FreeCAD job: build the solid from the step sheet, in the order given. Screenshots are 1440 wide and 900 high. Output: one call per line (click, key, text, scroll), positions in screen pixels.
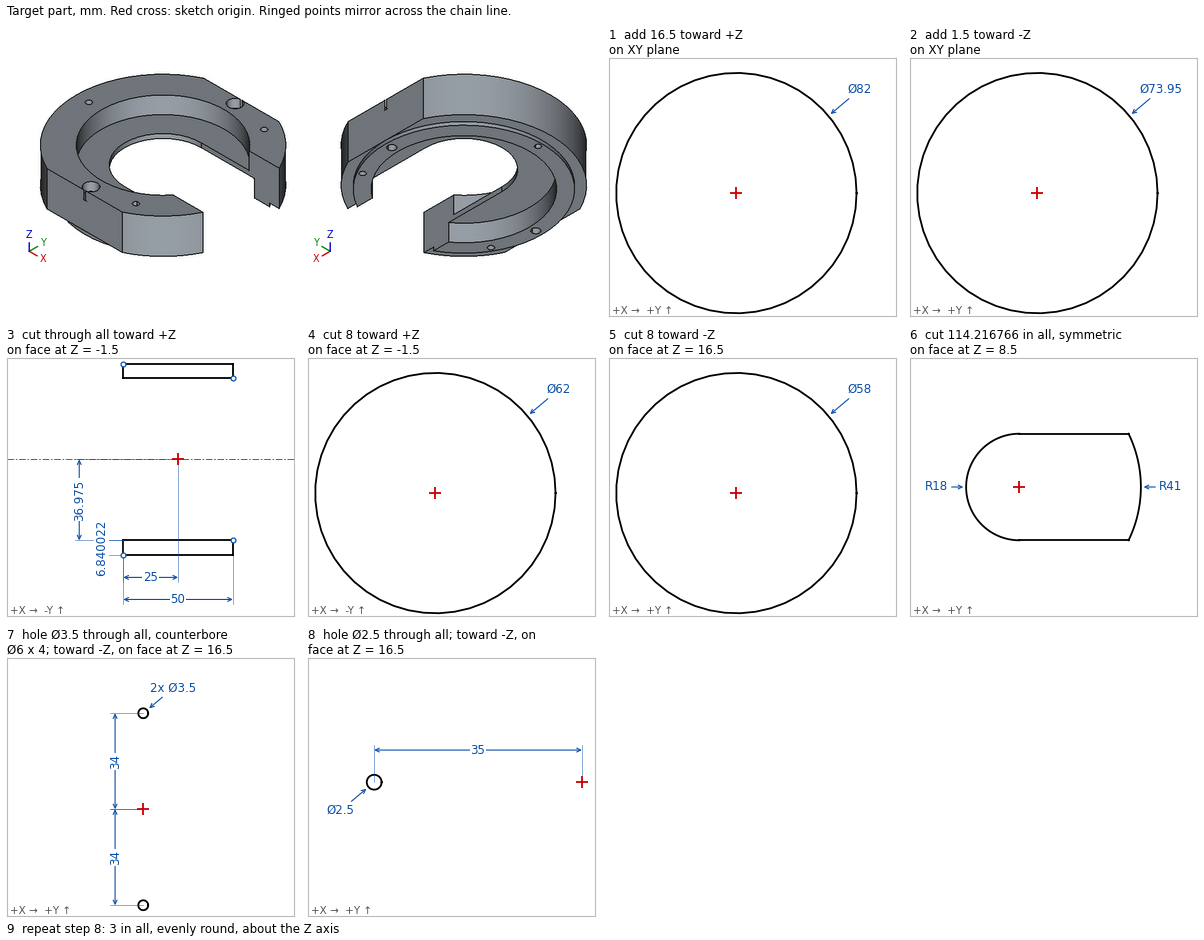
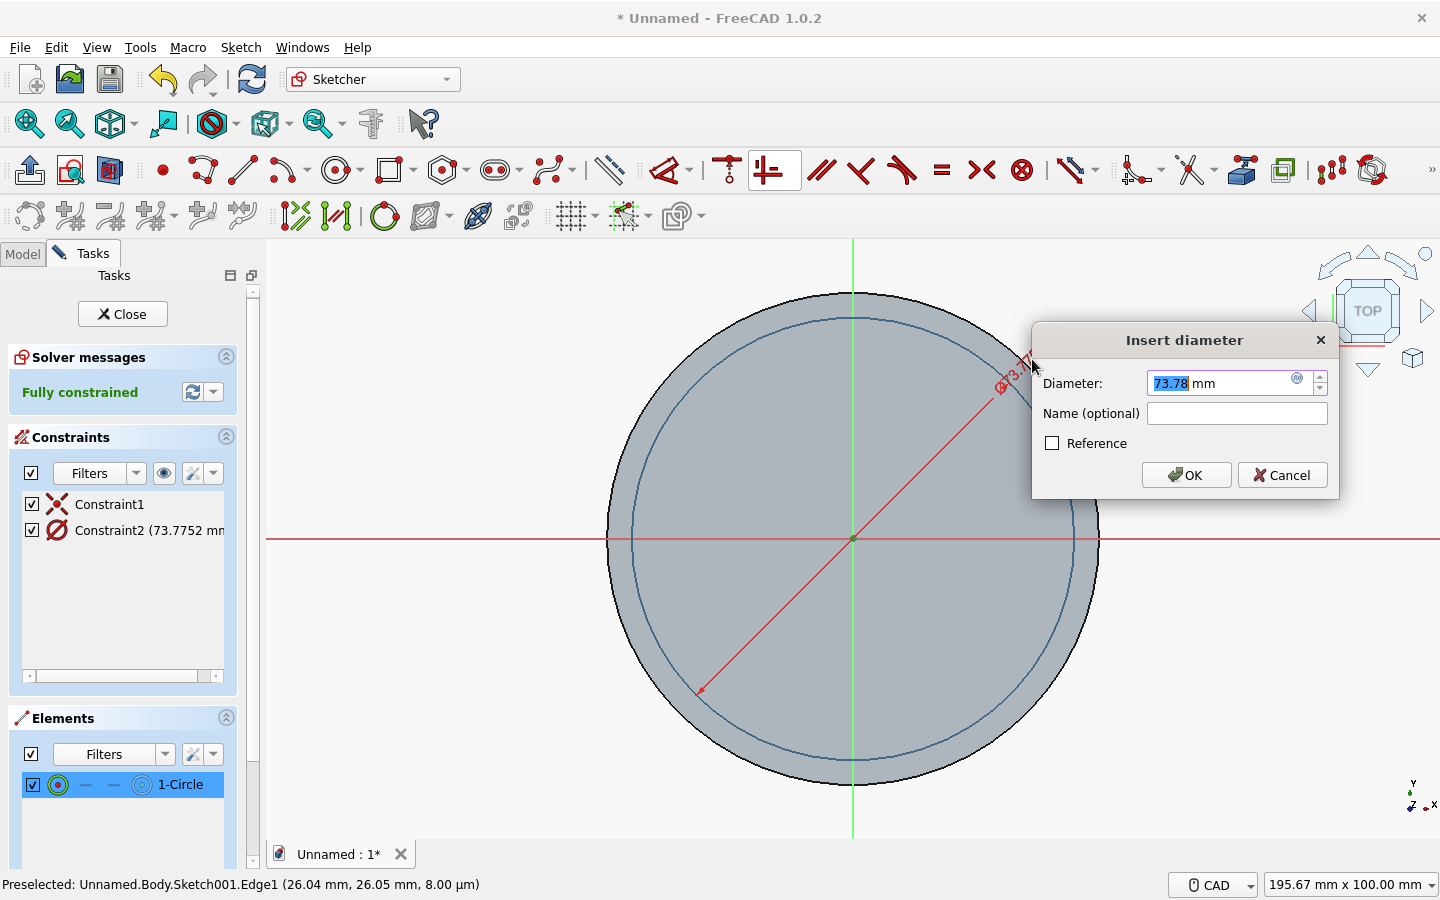
text(73.95)
key(Return)
key(Escape)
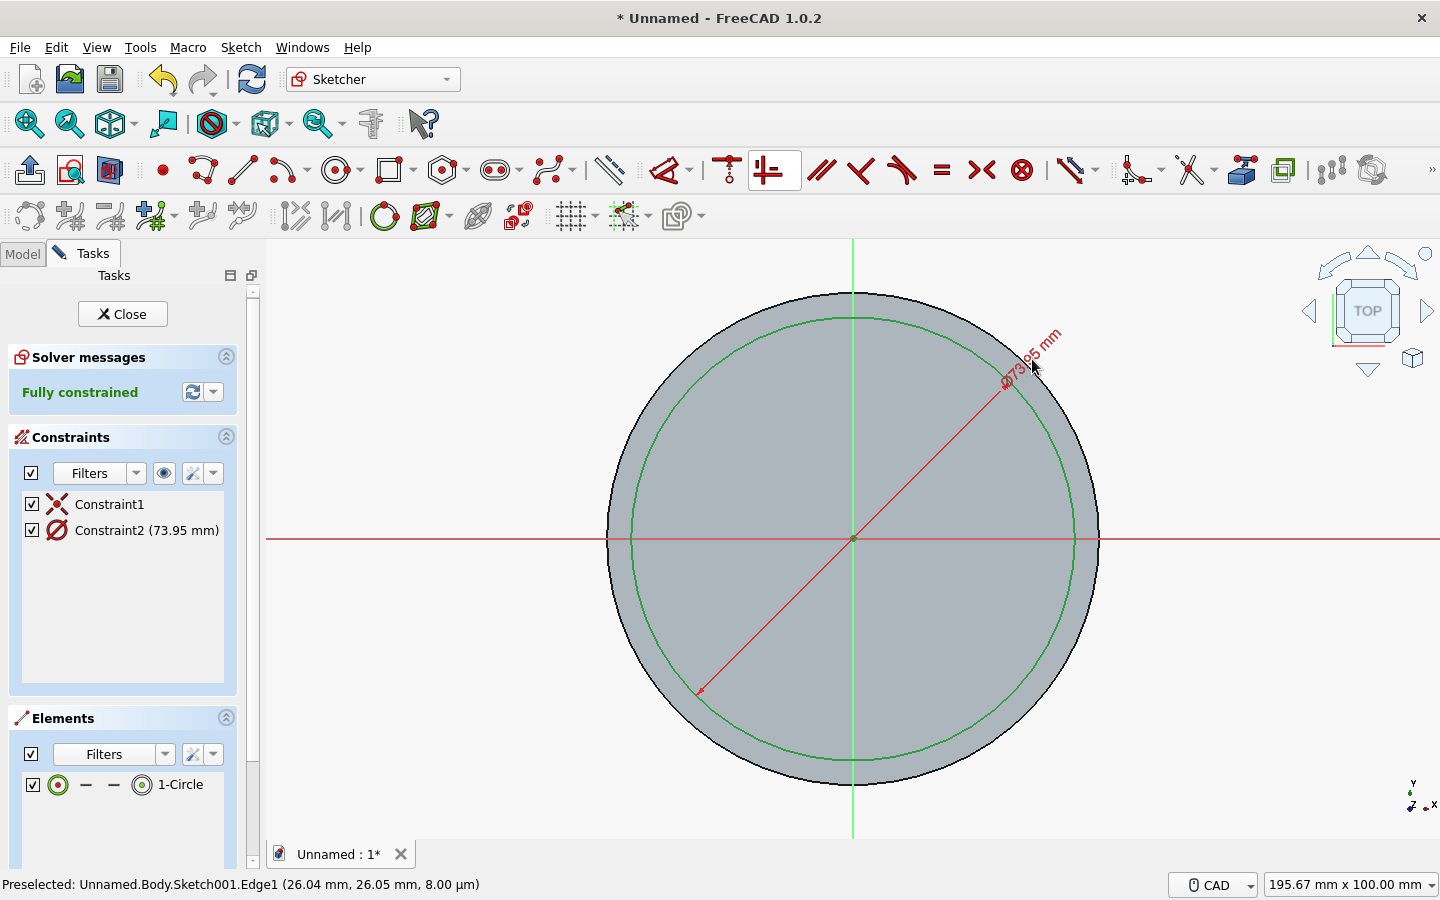
click(123, 314)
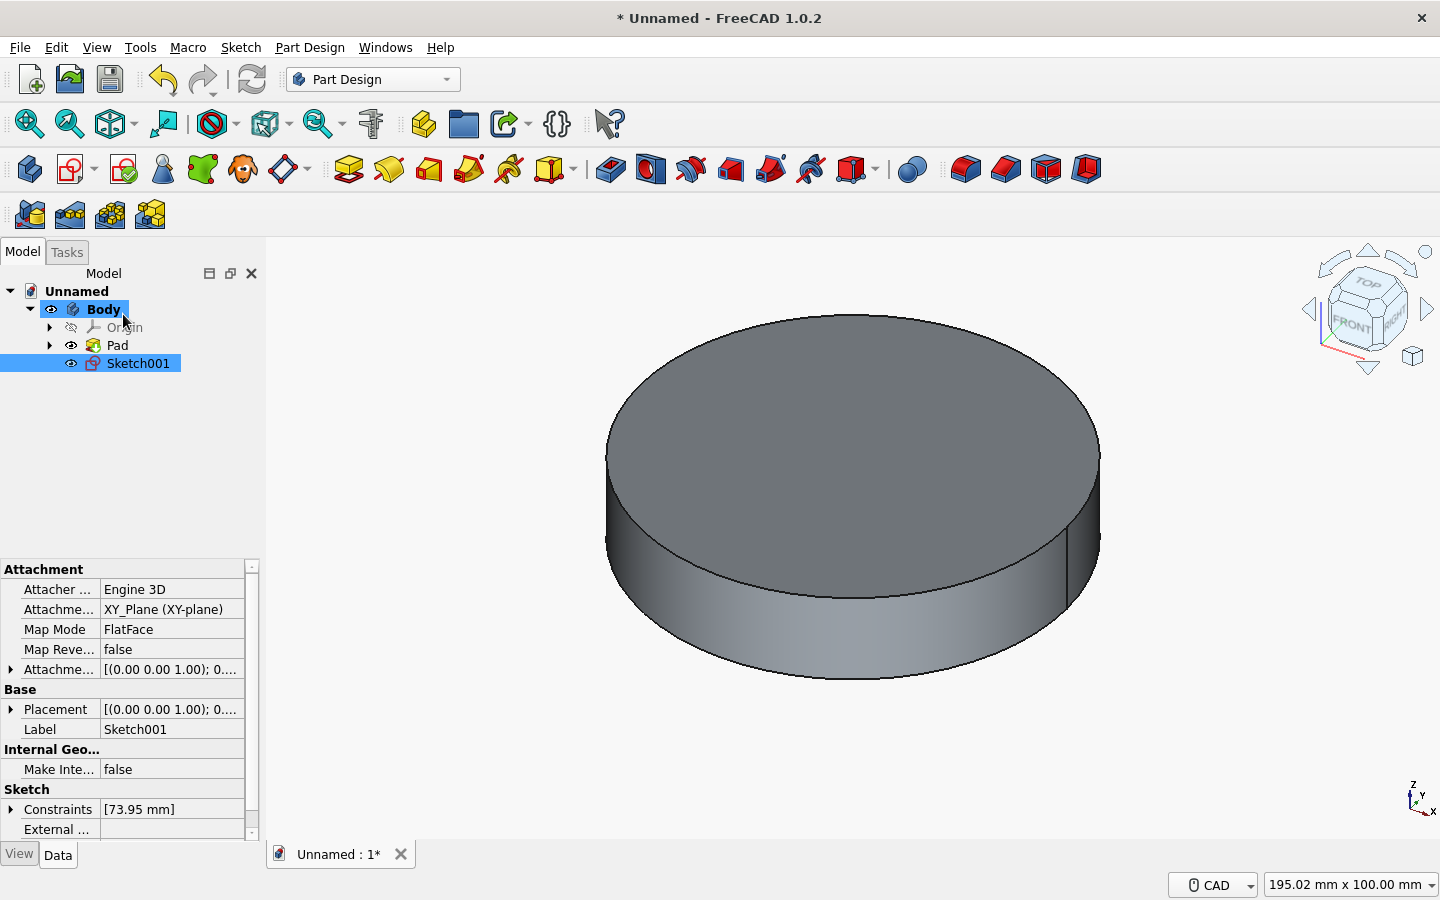
click(350, 170)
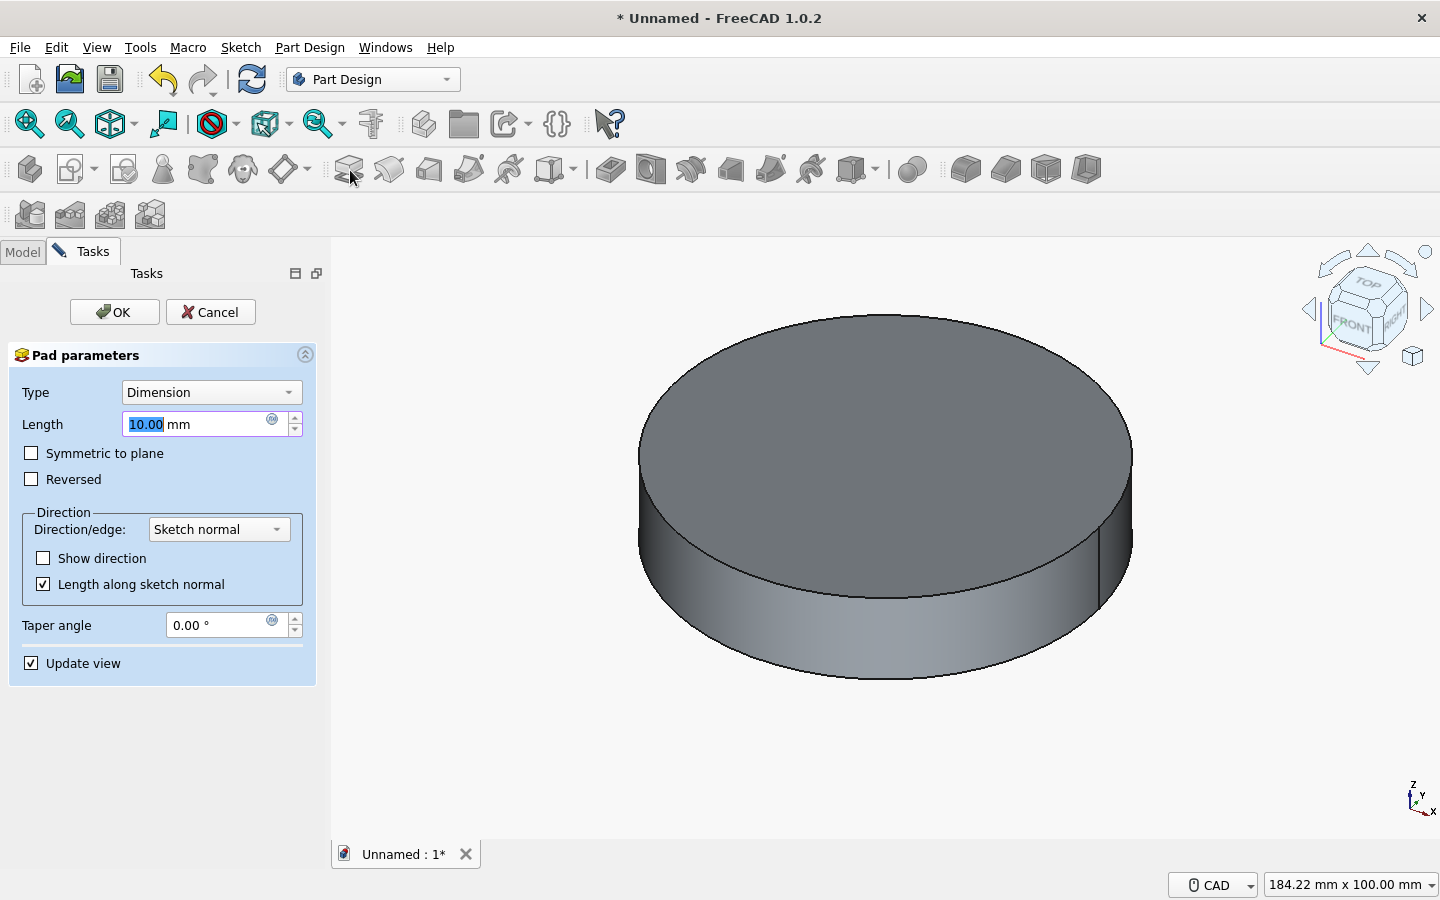
text(1.5)
key(Tab)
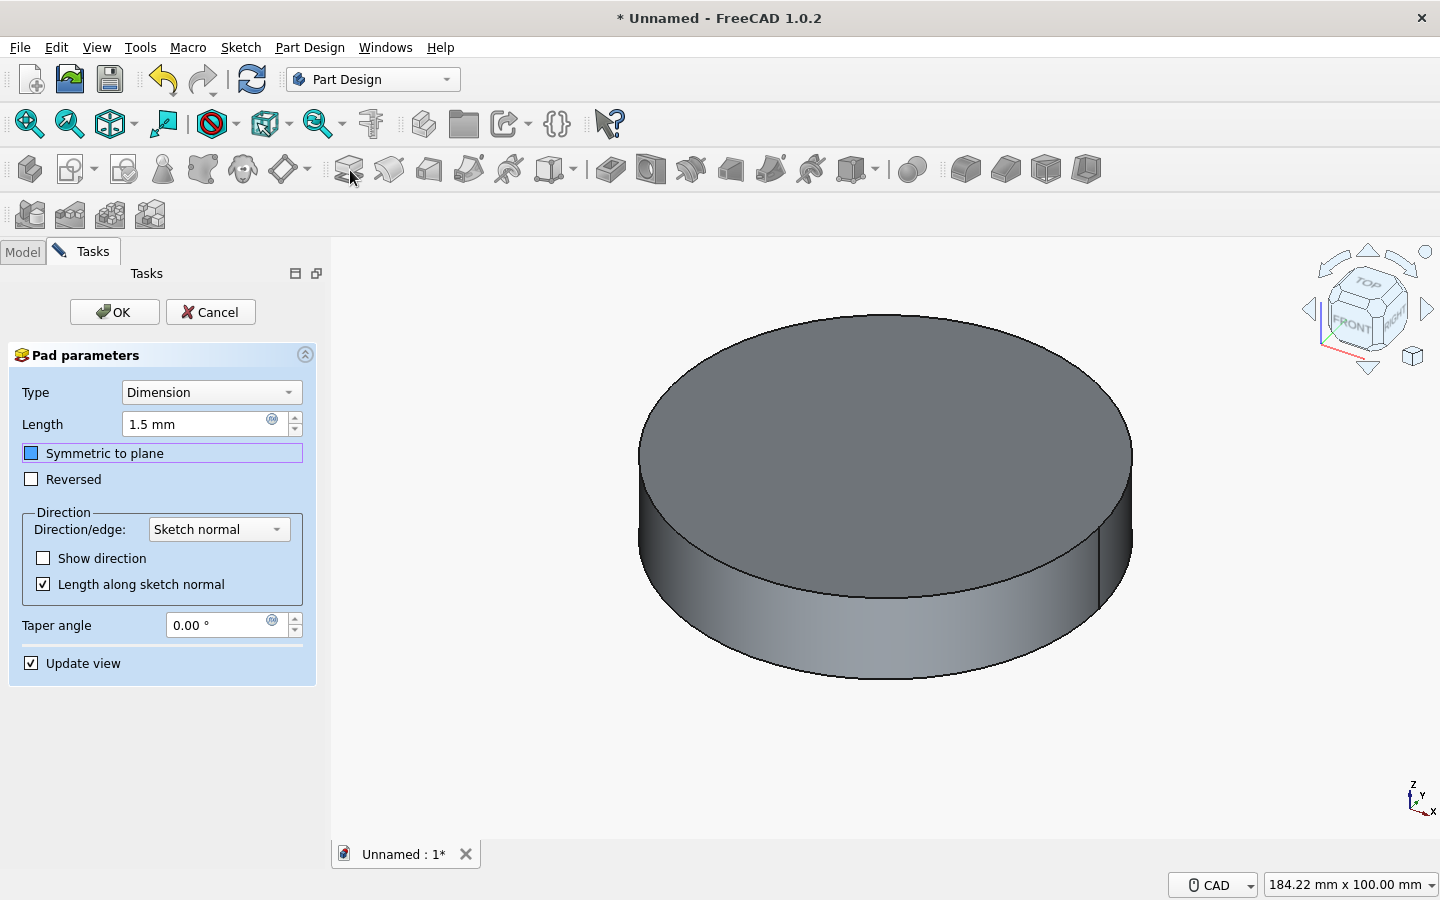
click(30, 479)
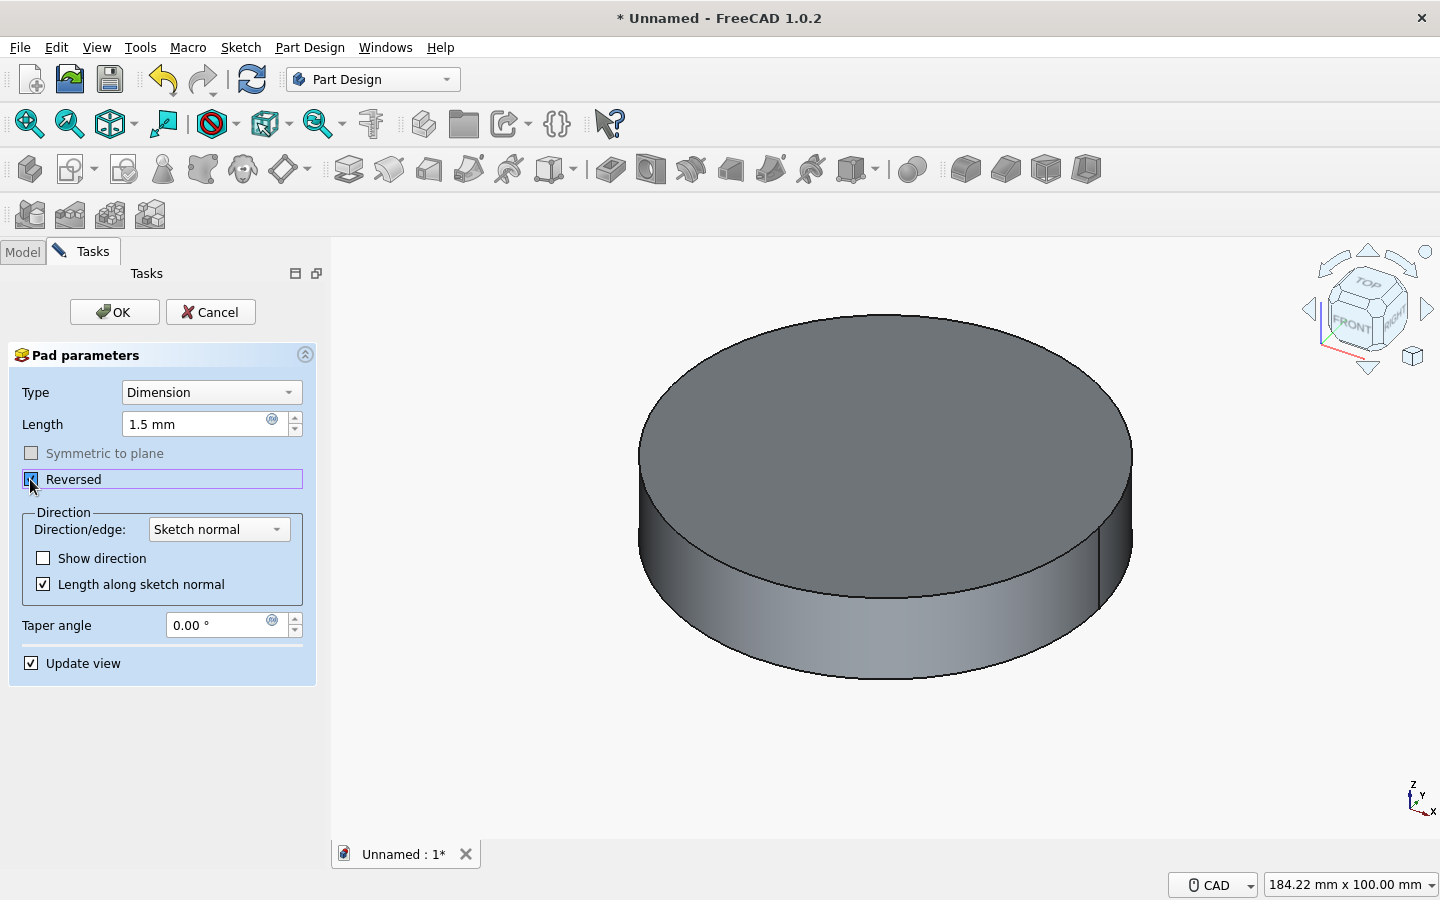
click(115, 312)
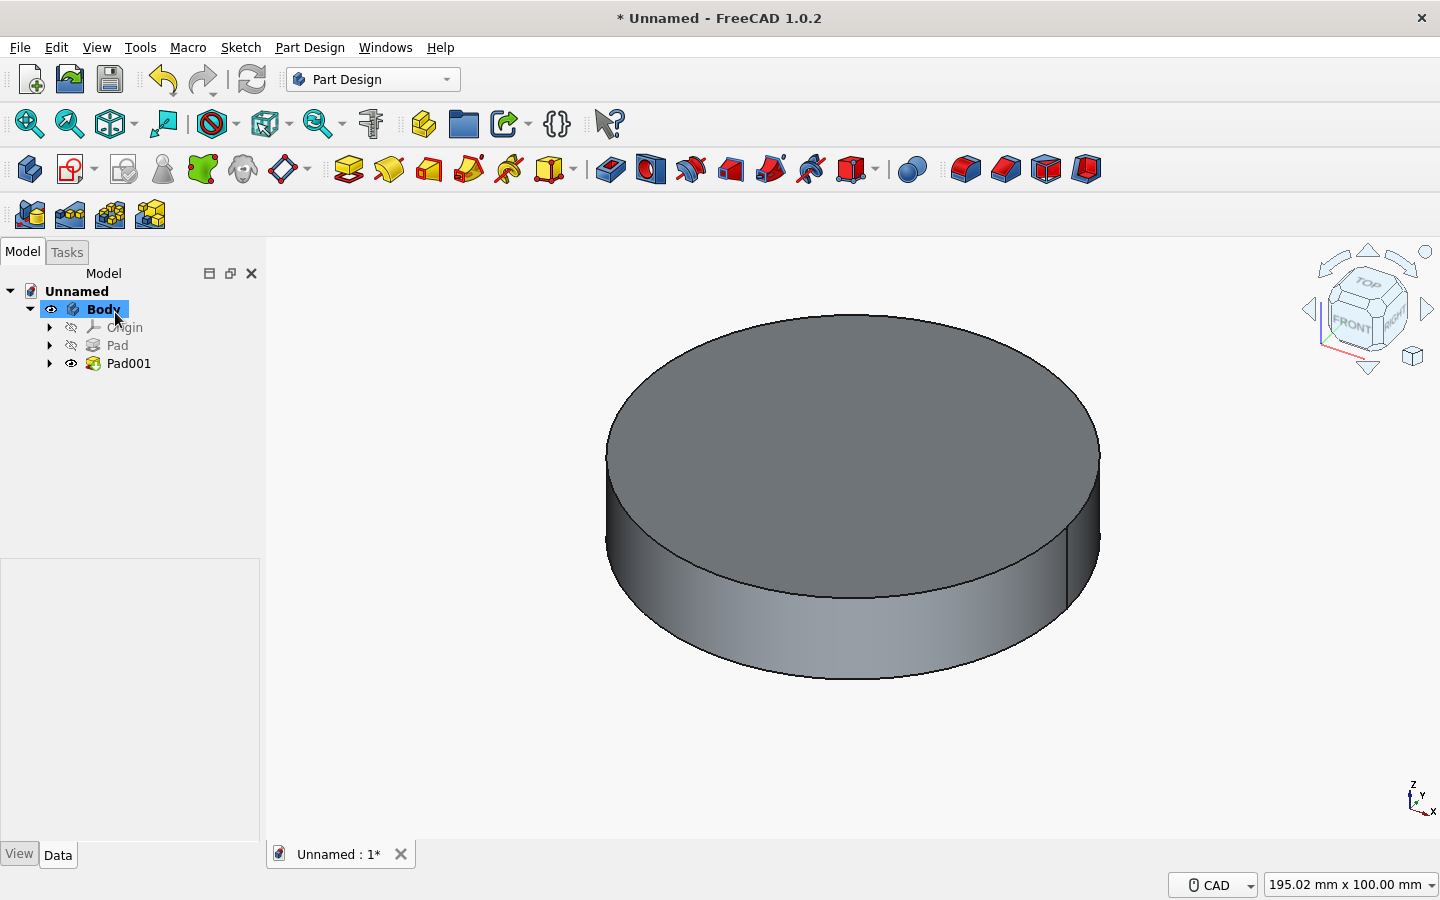
key(5)